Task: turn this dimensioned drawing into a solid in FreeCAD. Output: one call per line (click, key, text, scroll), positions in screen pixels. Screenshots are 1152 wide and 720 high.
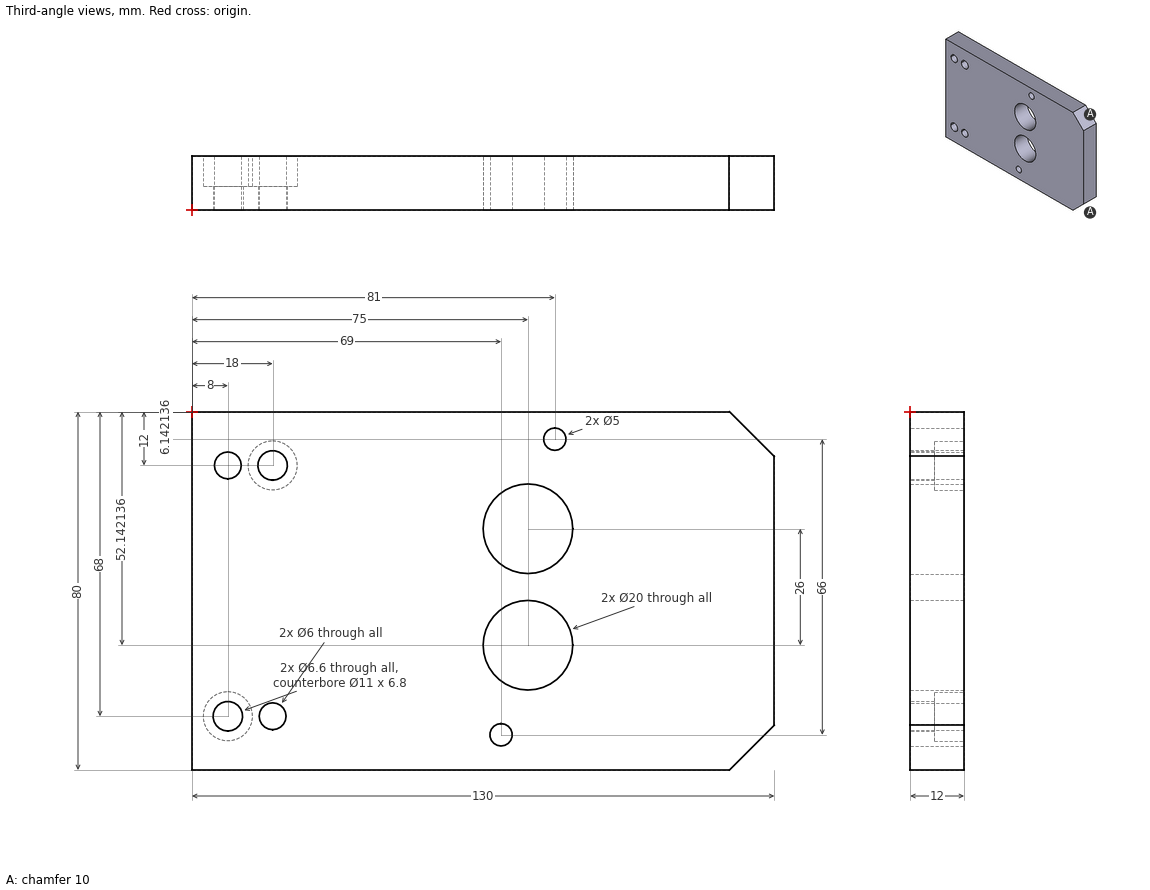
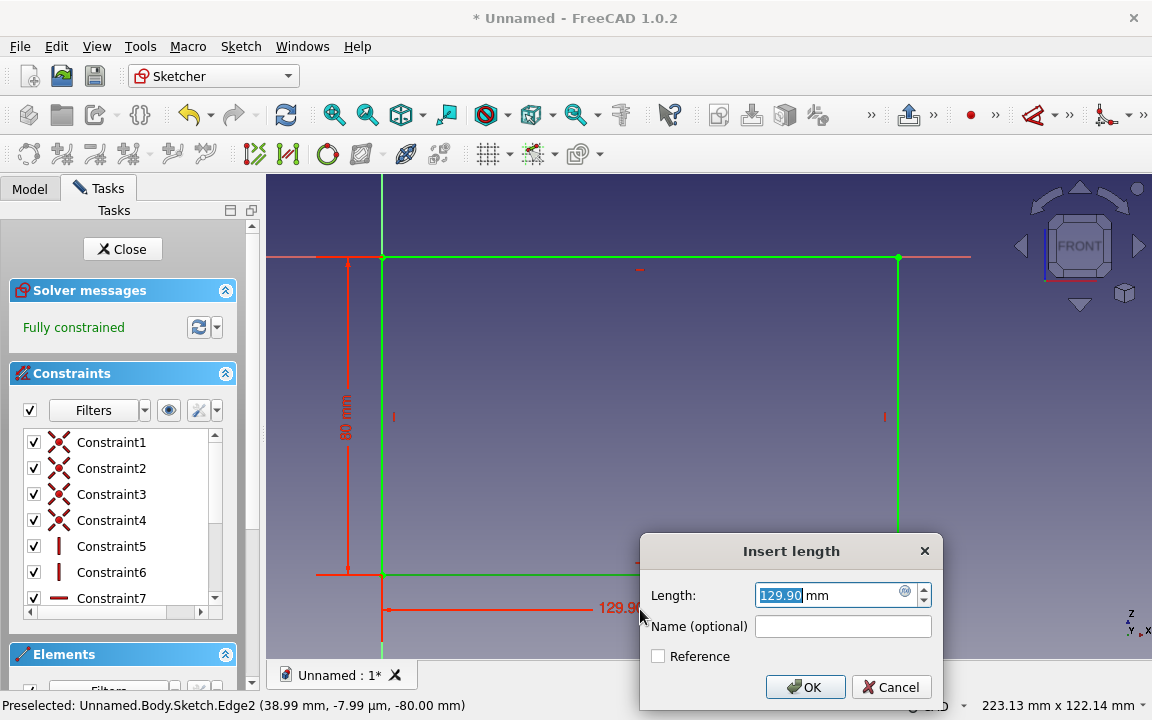
text(130)
key(Return)
key(Escape)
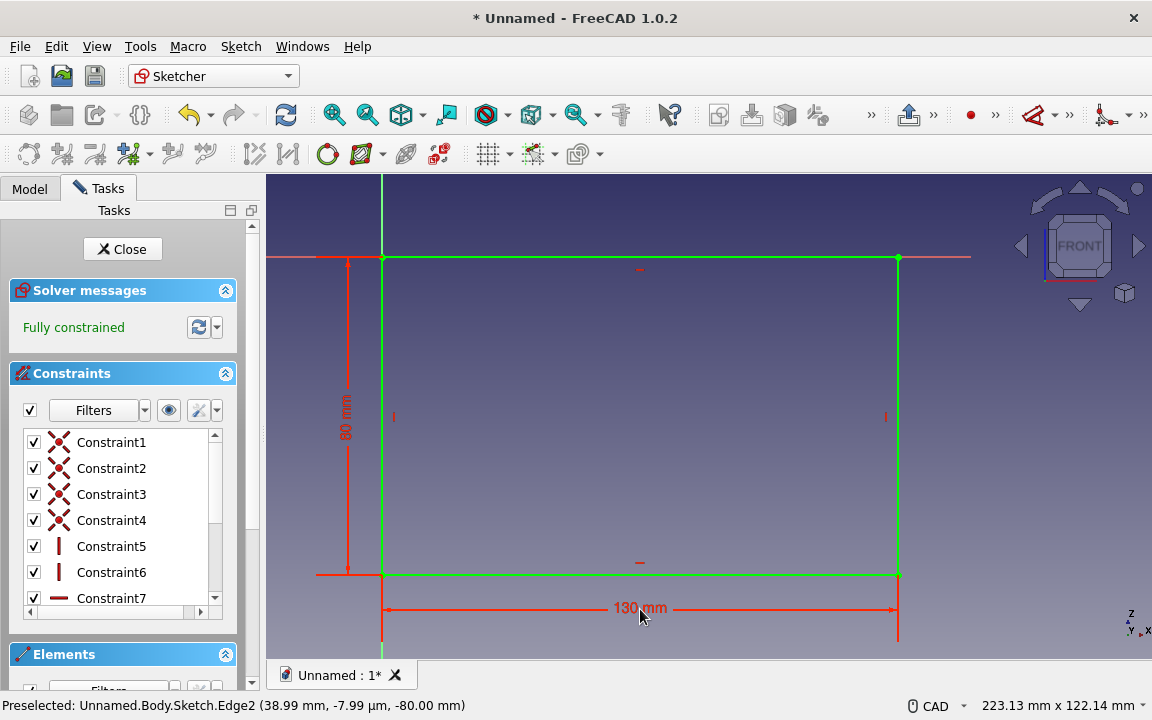
click(123, 249)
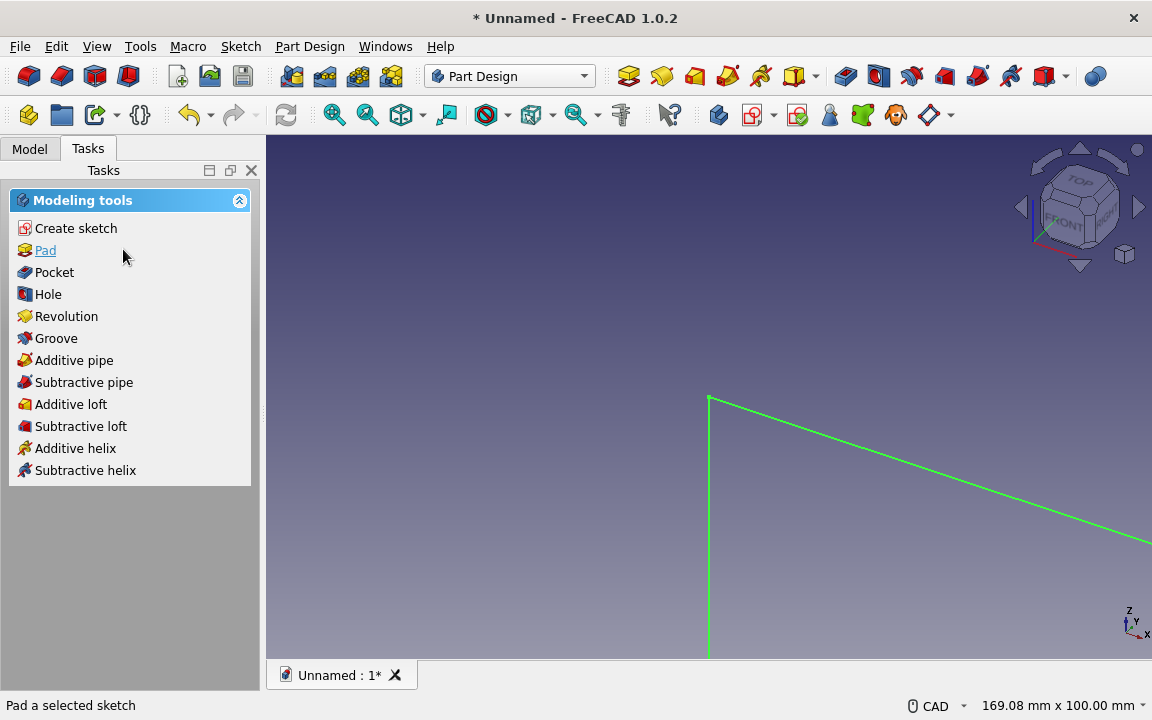
click(629, 76)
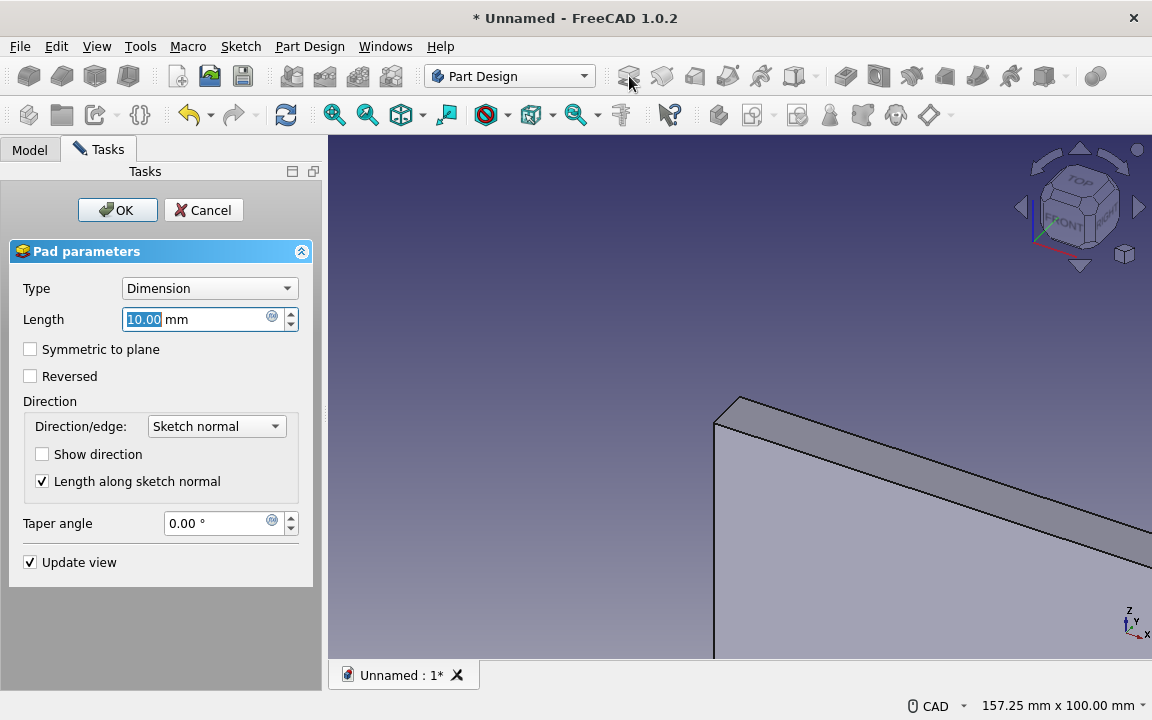
text(12)
key(Tab)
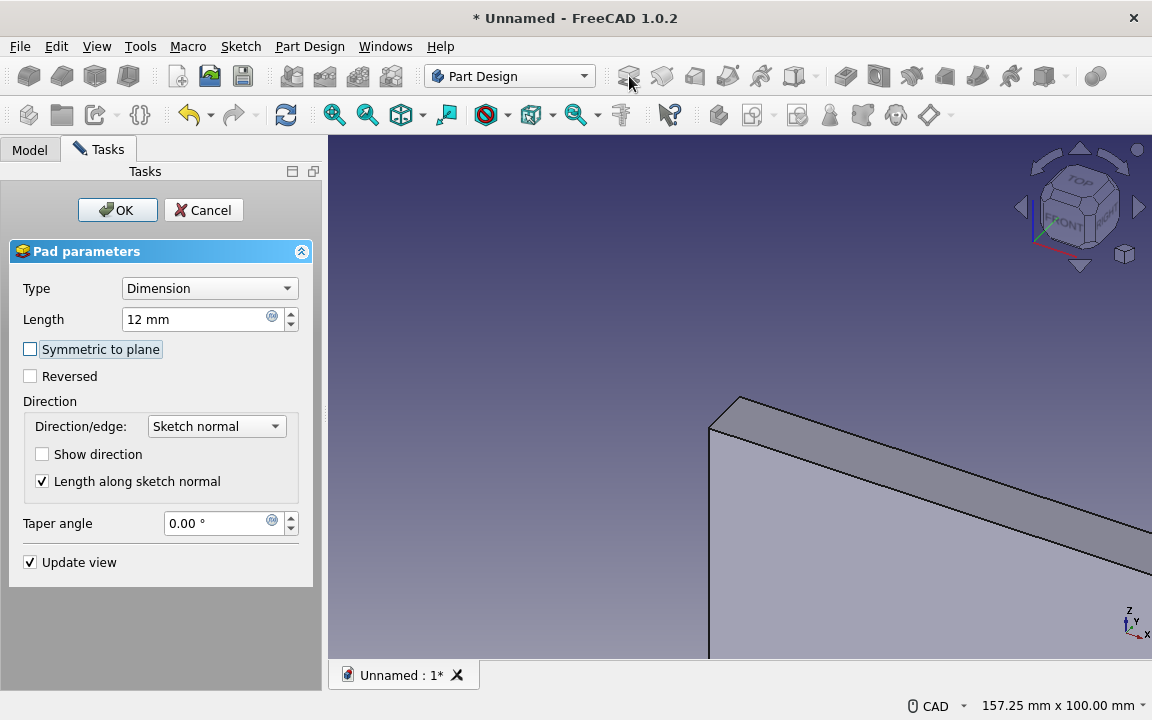
click(31, 376)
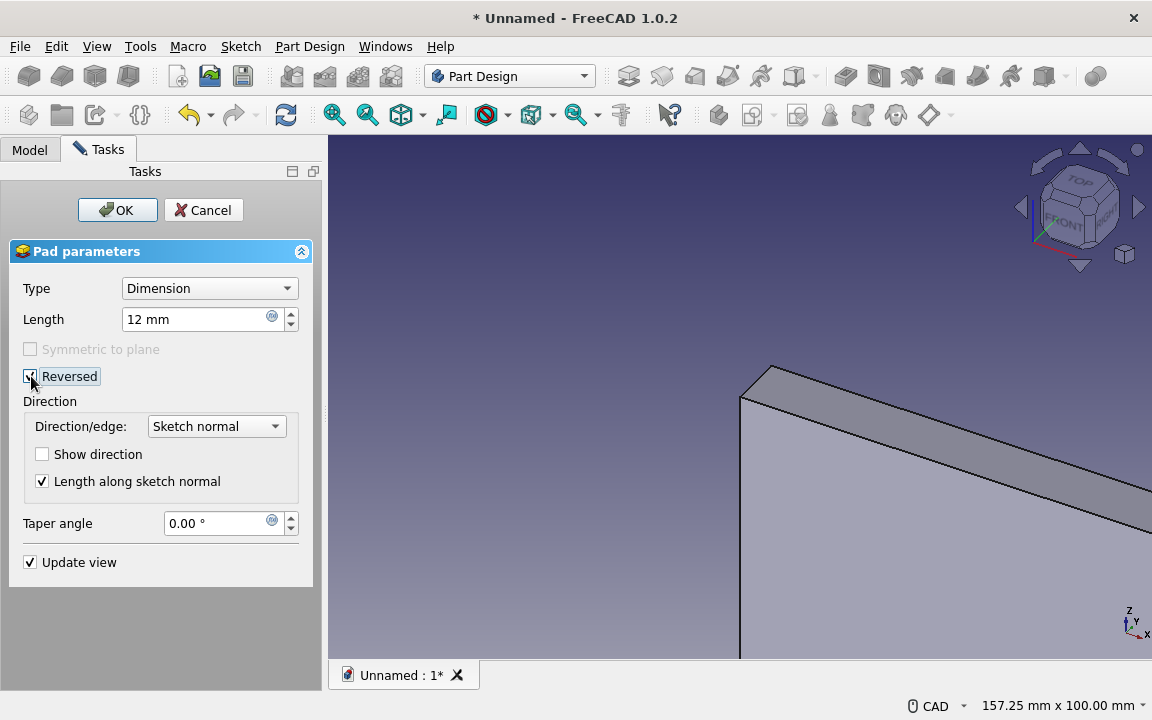
click(118, 210)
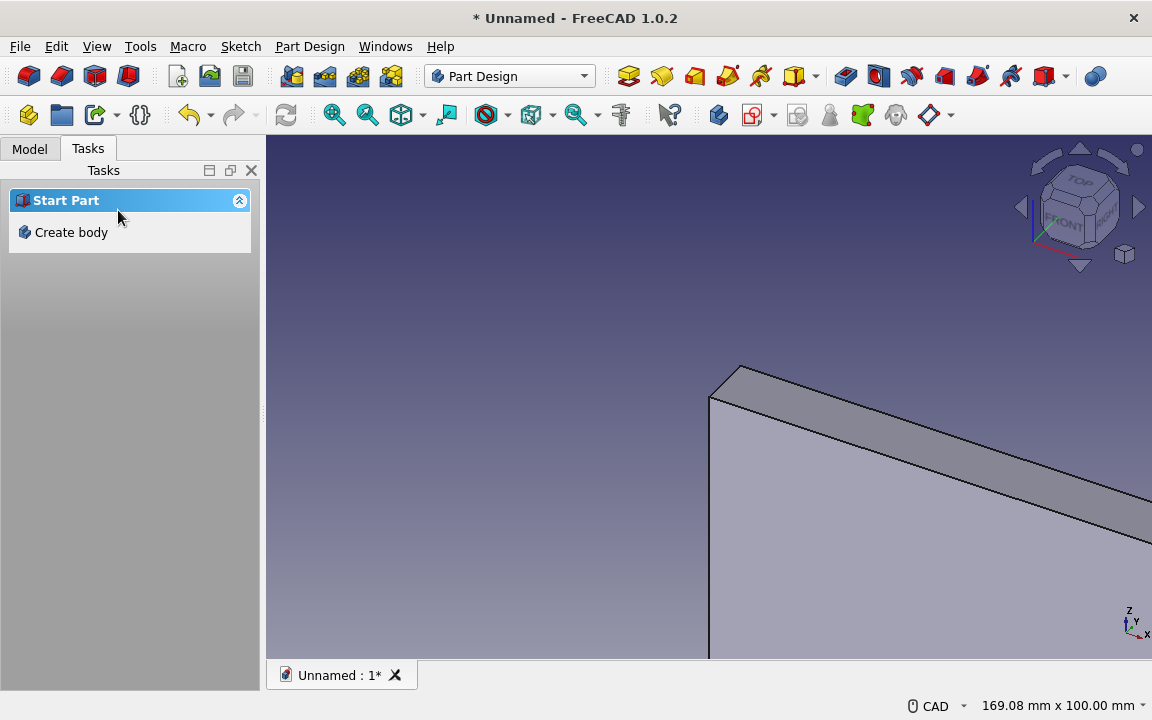
click(335, 116)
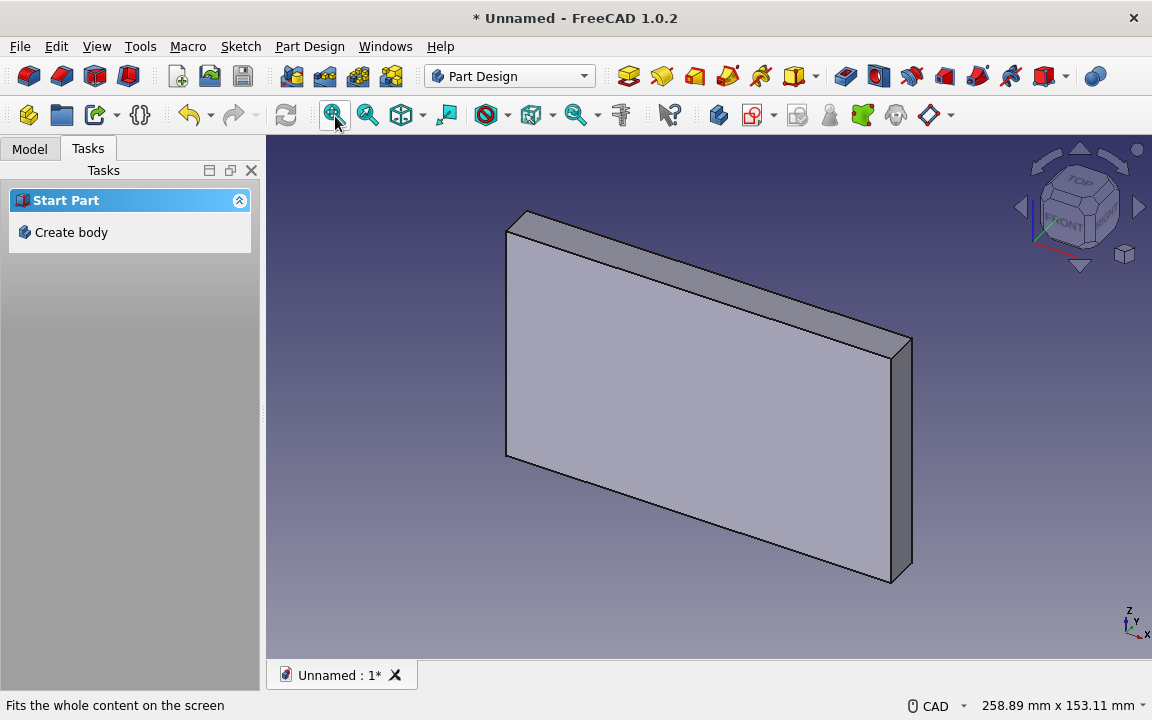
click(902, 348)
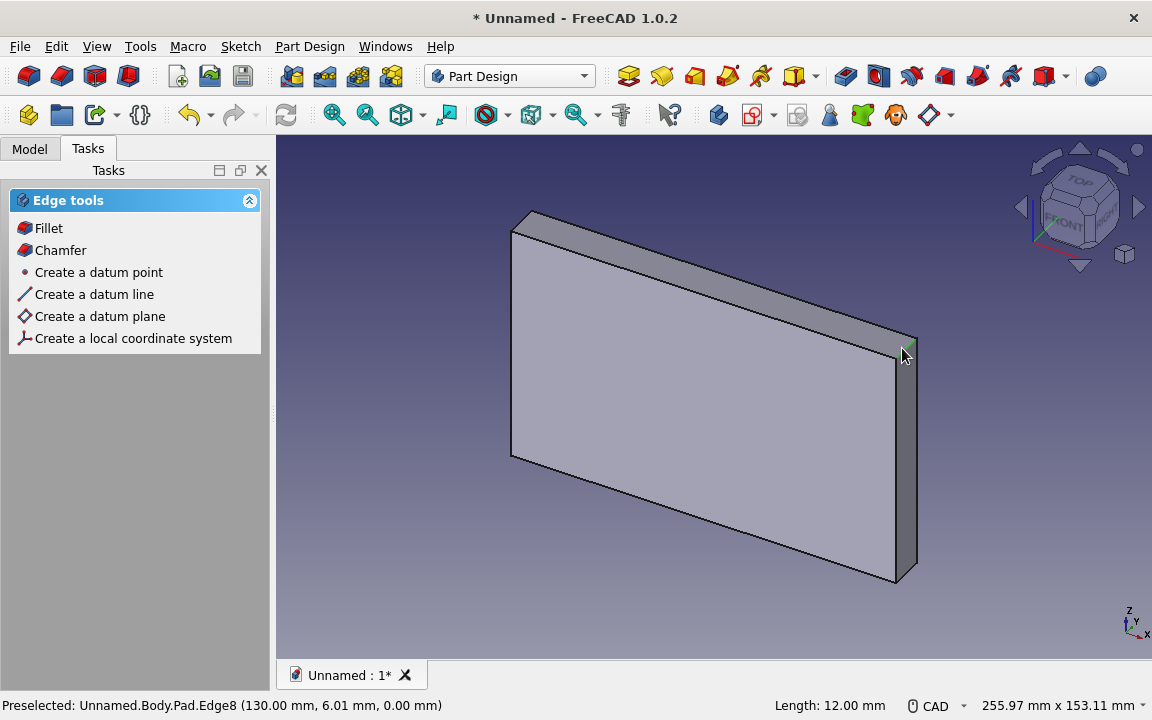
key(0)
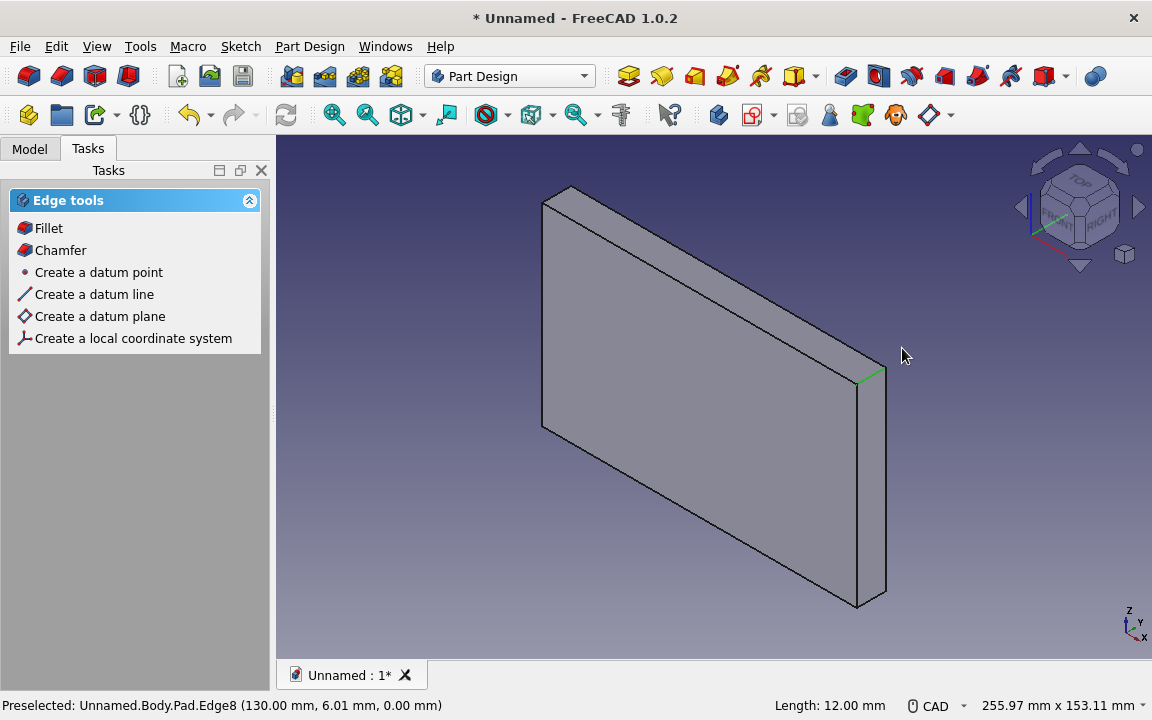
key(2)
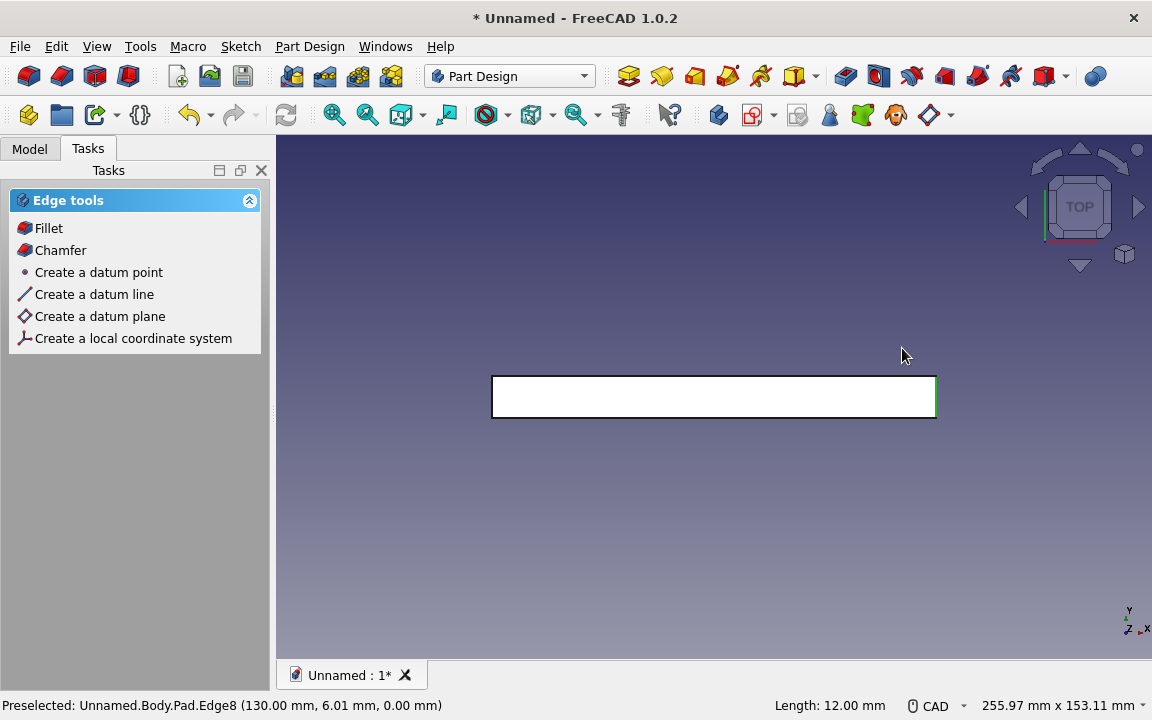
key(1)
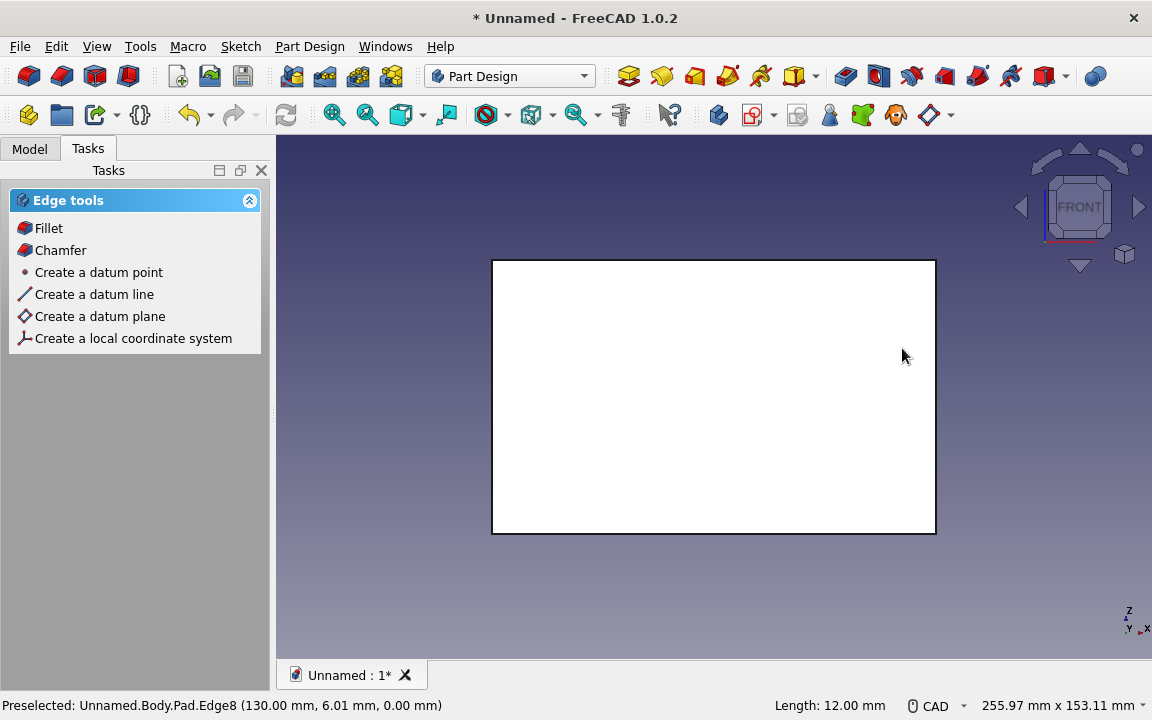
key(3)